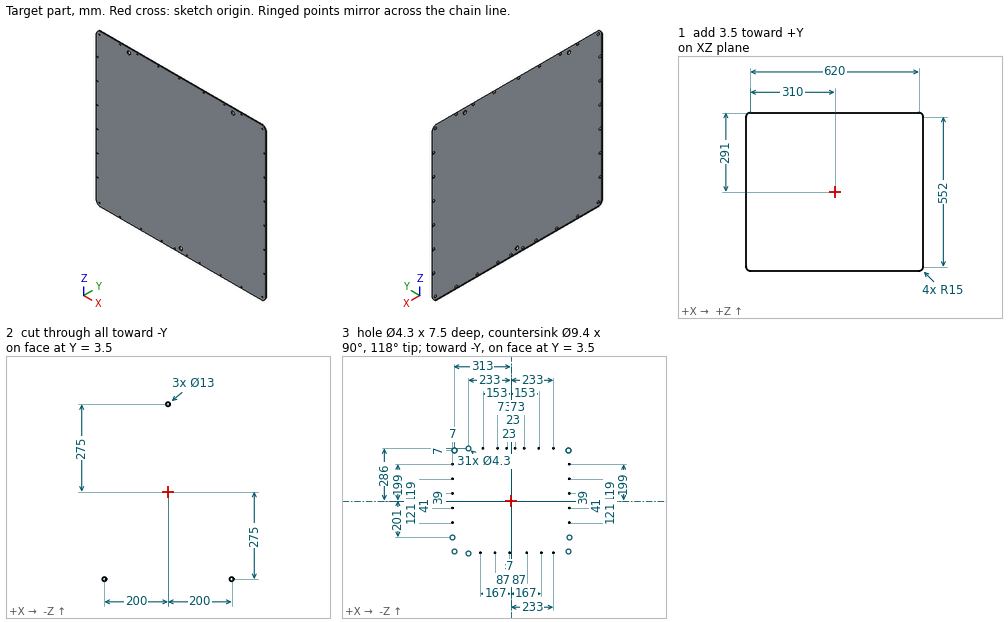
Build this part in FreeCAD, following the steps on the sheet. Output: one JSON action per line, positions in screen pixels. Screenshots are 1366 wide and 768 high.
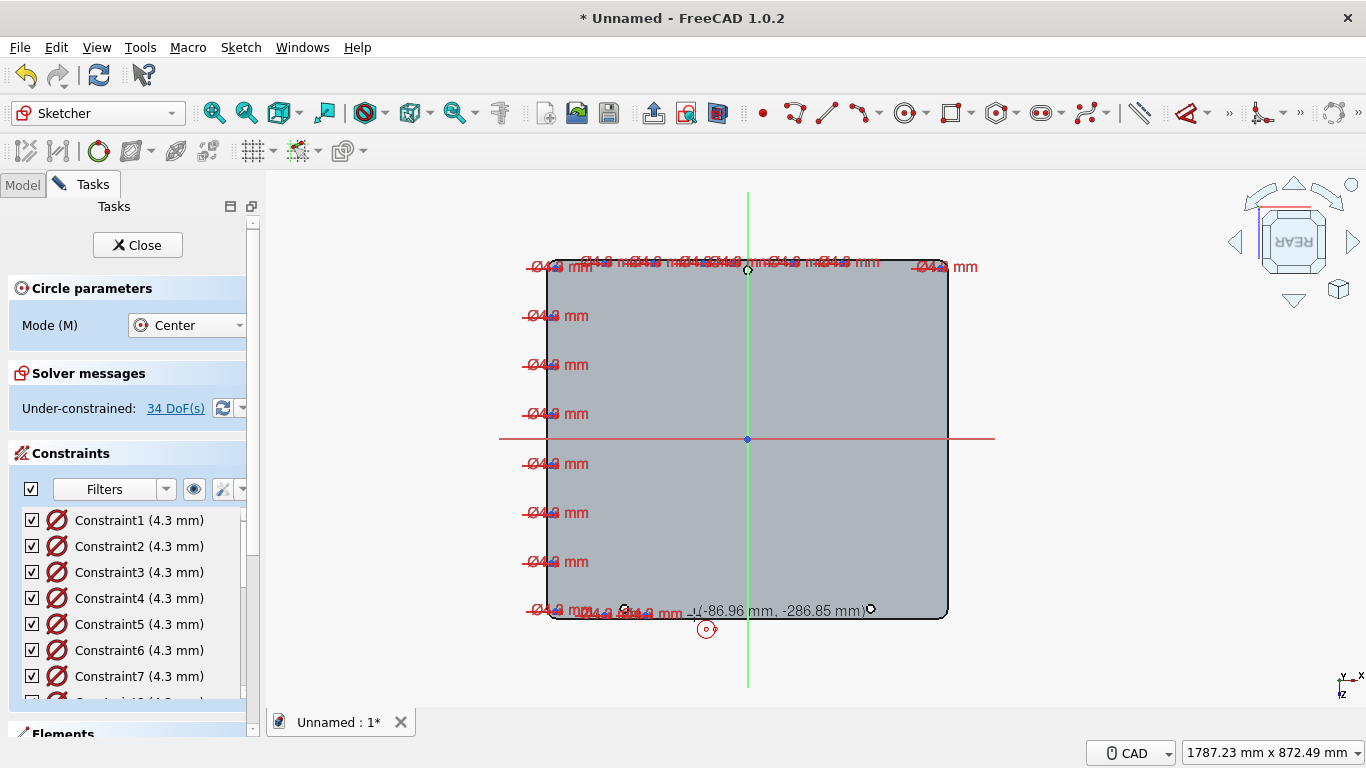
{"action": "left_click", "coordinate": [694, 615]}
{"action": "mouse_move", "coordinate": [695, 615]}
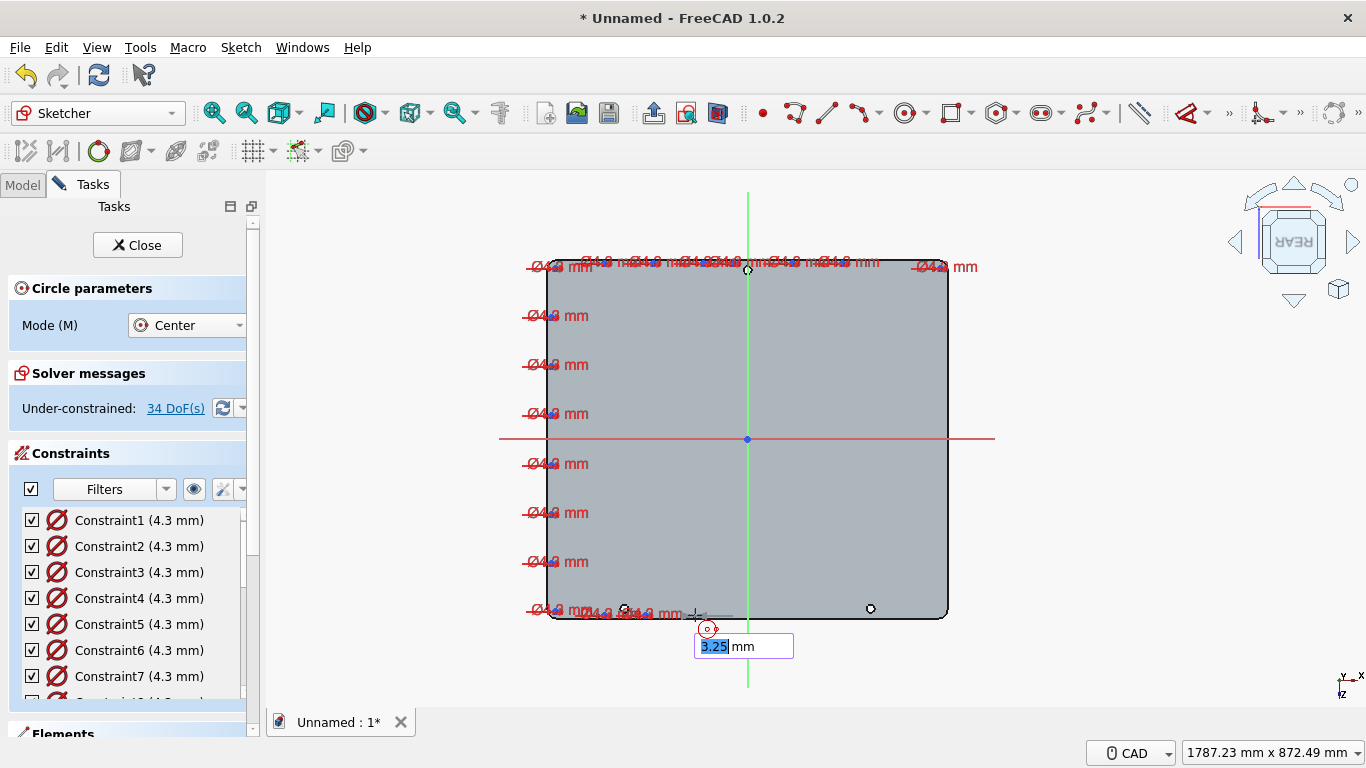
{"action": "type", "text": "4.3"}
{"action": "key", "text": "Return"}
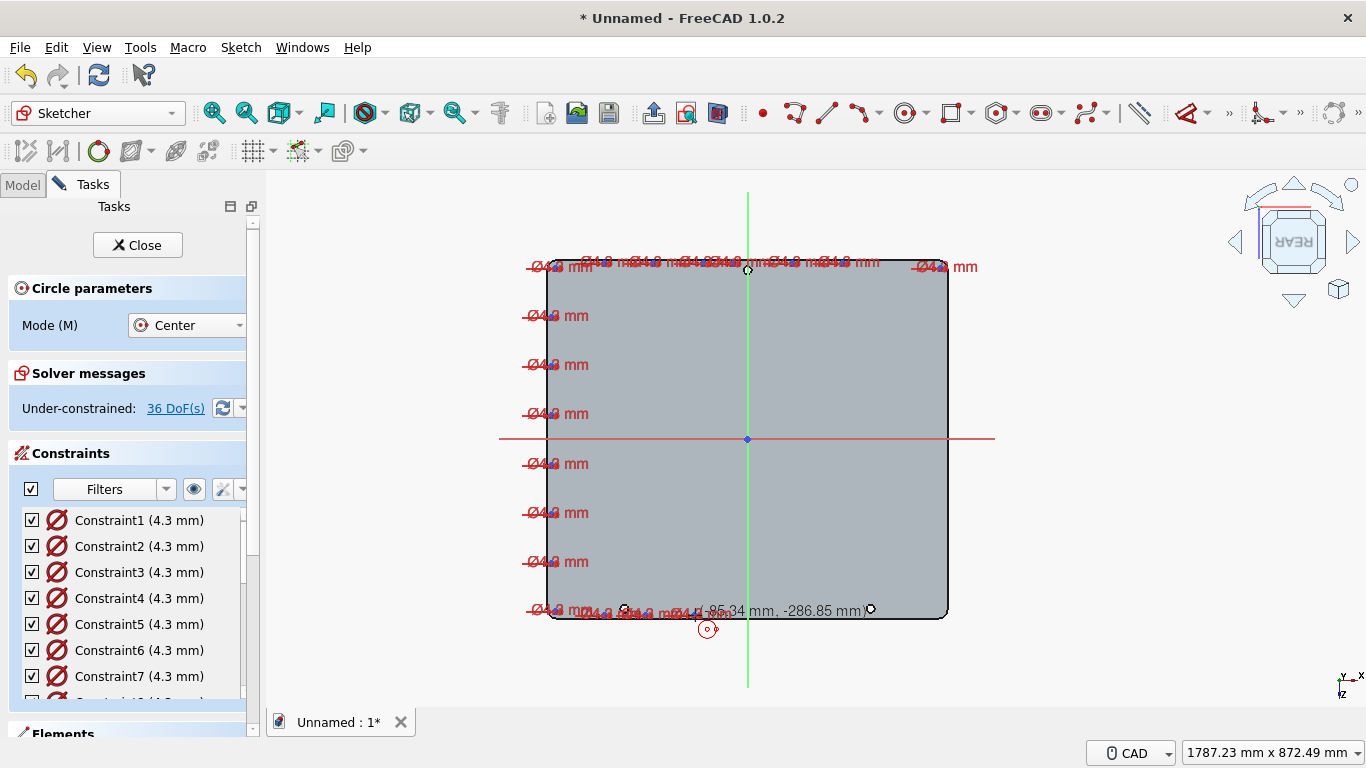
{"action": "scroll", "coordinate": [743, 615], "scroll_direction": "up", "scroll_amount": 15}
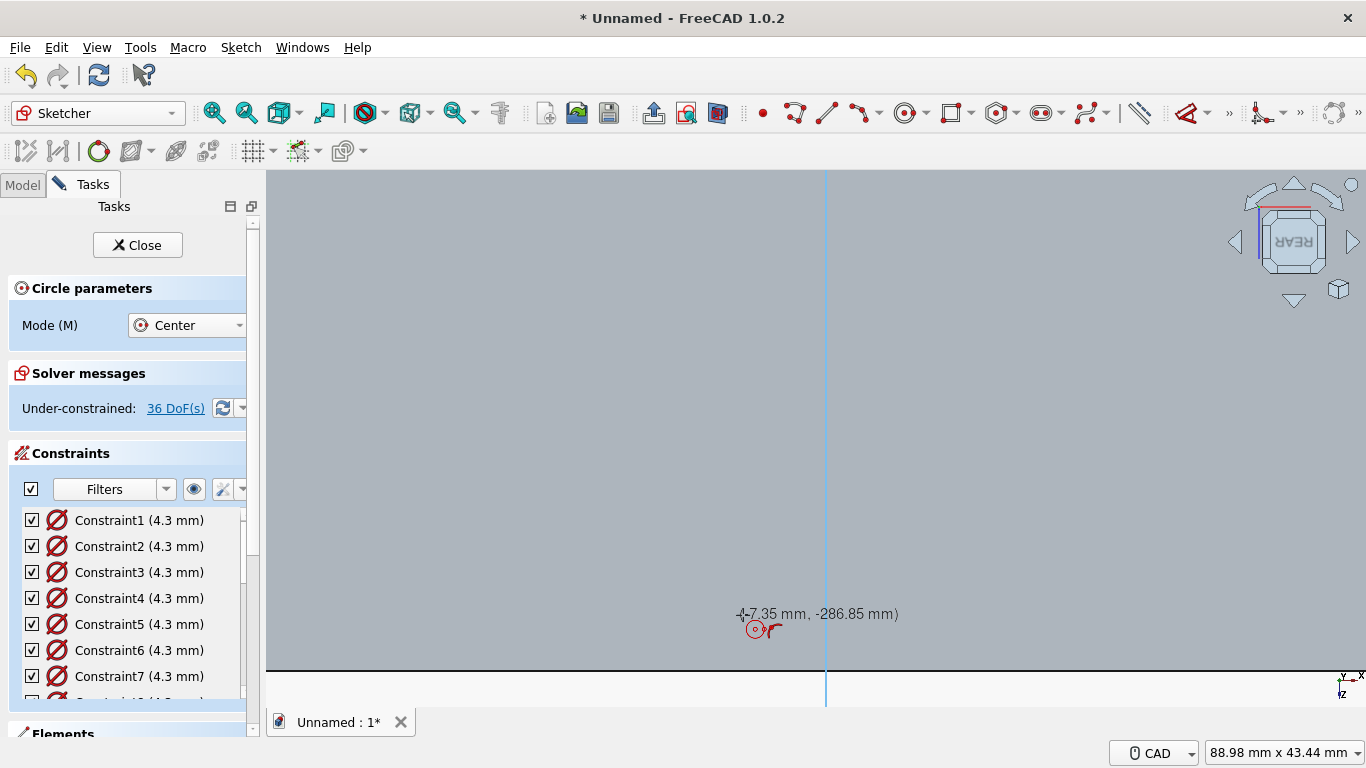
{"action": "scroll", "coordinate": [743, 615], "scroll_direction": "down", "scroll_amount": 15}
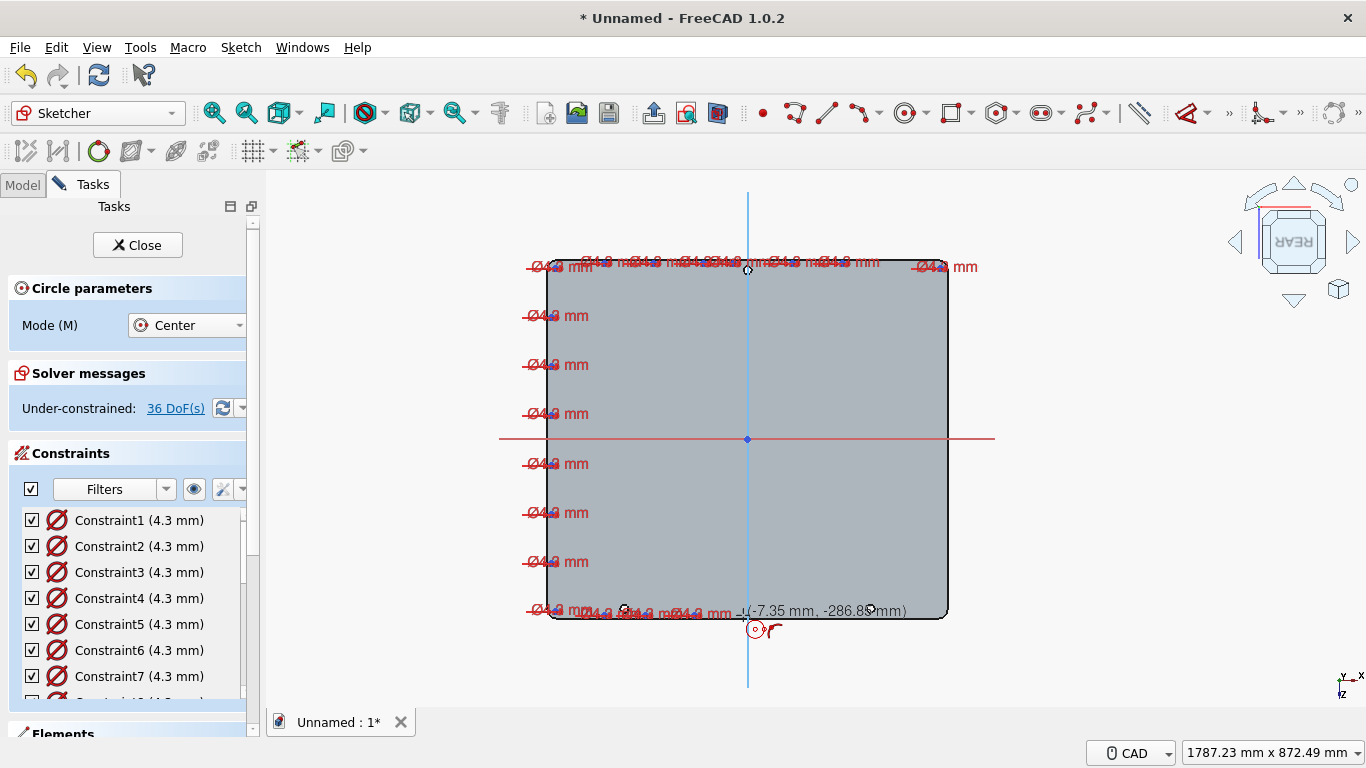
{"action": "scroll", "coordinate": [743, 615], "scroll_direction": "up", "scroll_amount": 7}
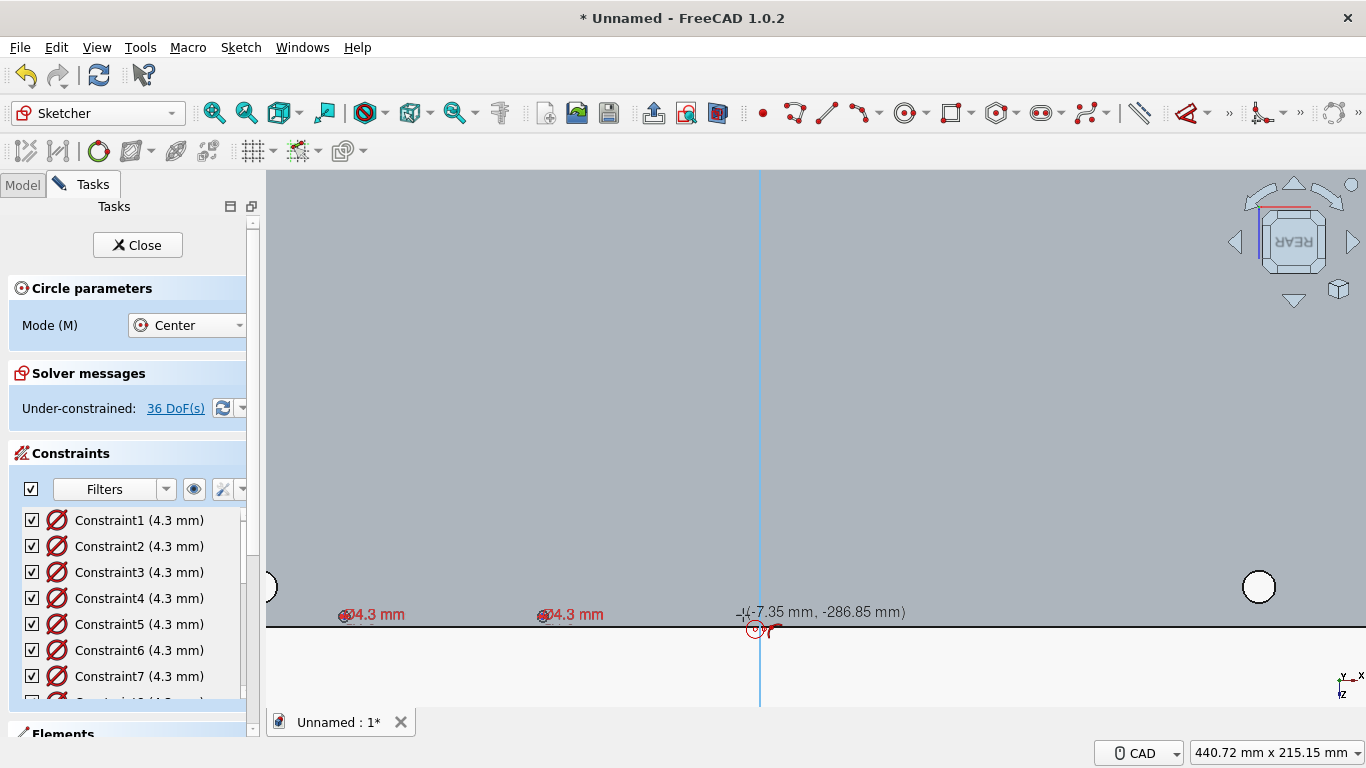
{"action": "left_click", "coordinate": [743, 614]}
{"action": "mouse_move", "coordinate": [739, 611]}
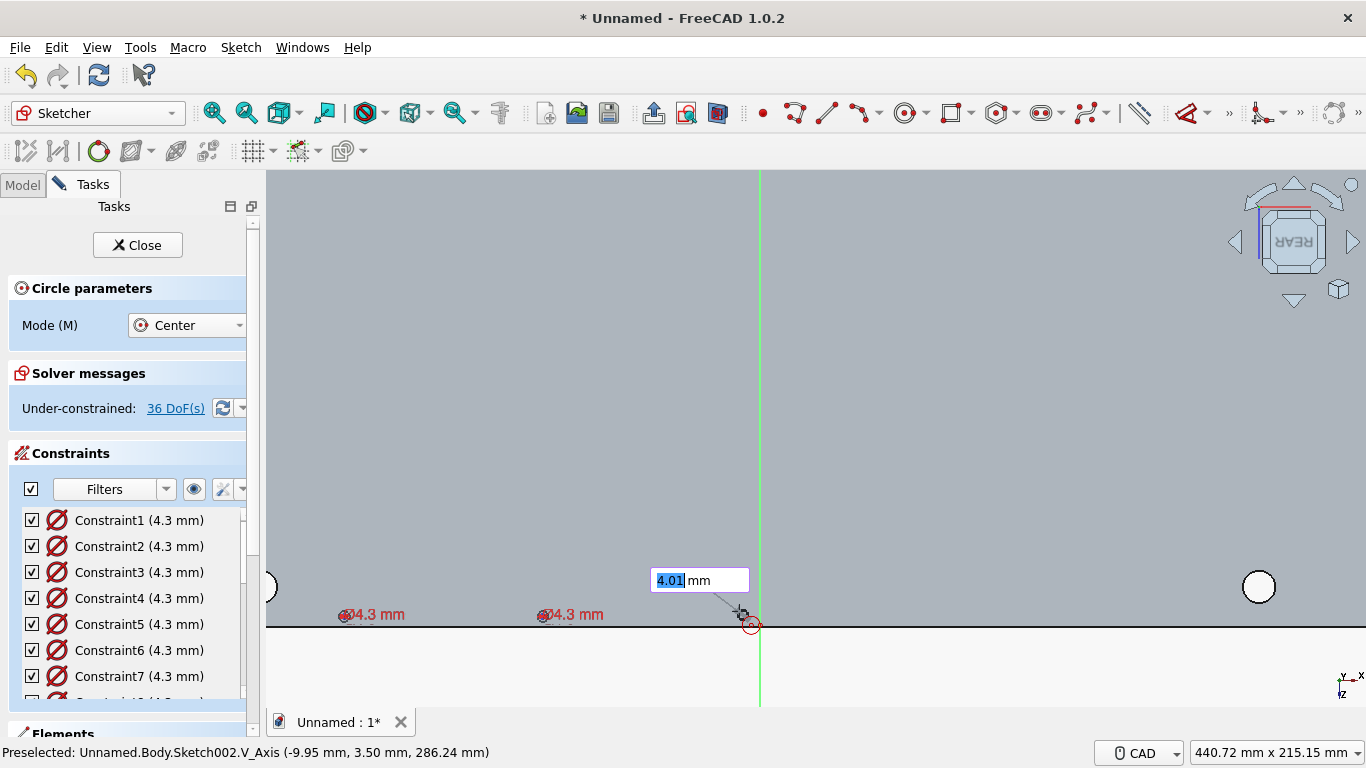
{"action": "type", "text": "4.3"}
{"action": "key", "text": "Return"}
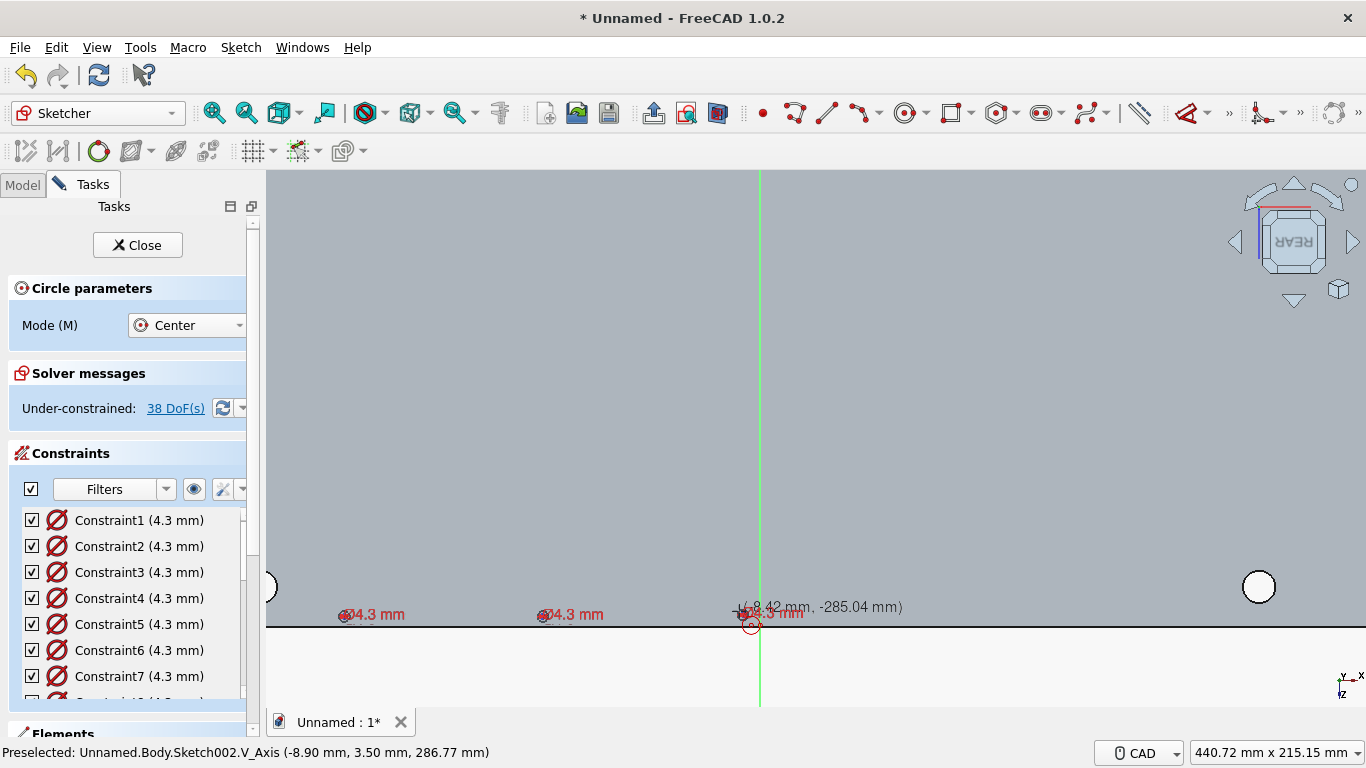
{"action": "scroll", "coordinate": [977, 614], "scroll_direction": "up", "scroll_amount": 8}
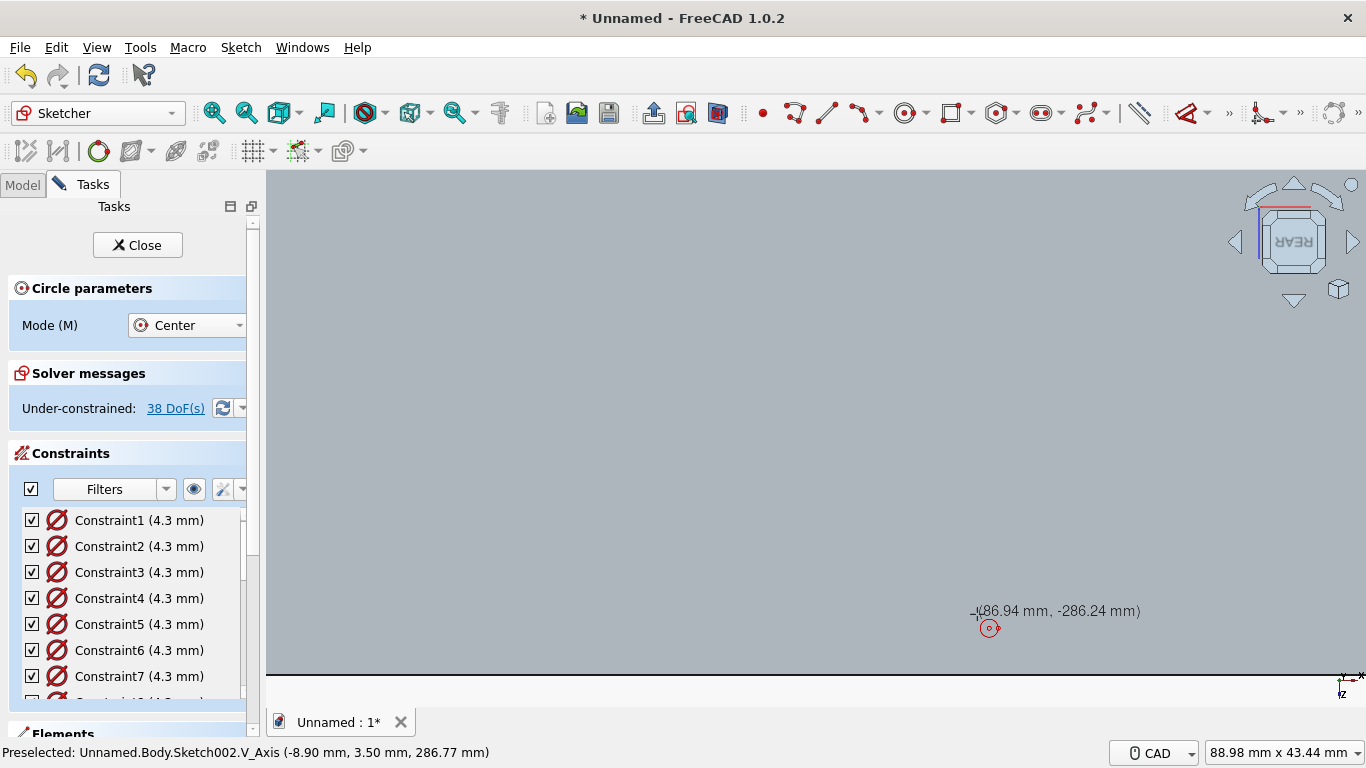
{"action": "scroll", "coordinate": [792, 615], "scroll_direction": "down", "scroll_amount": 15}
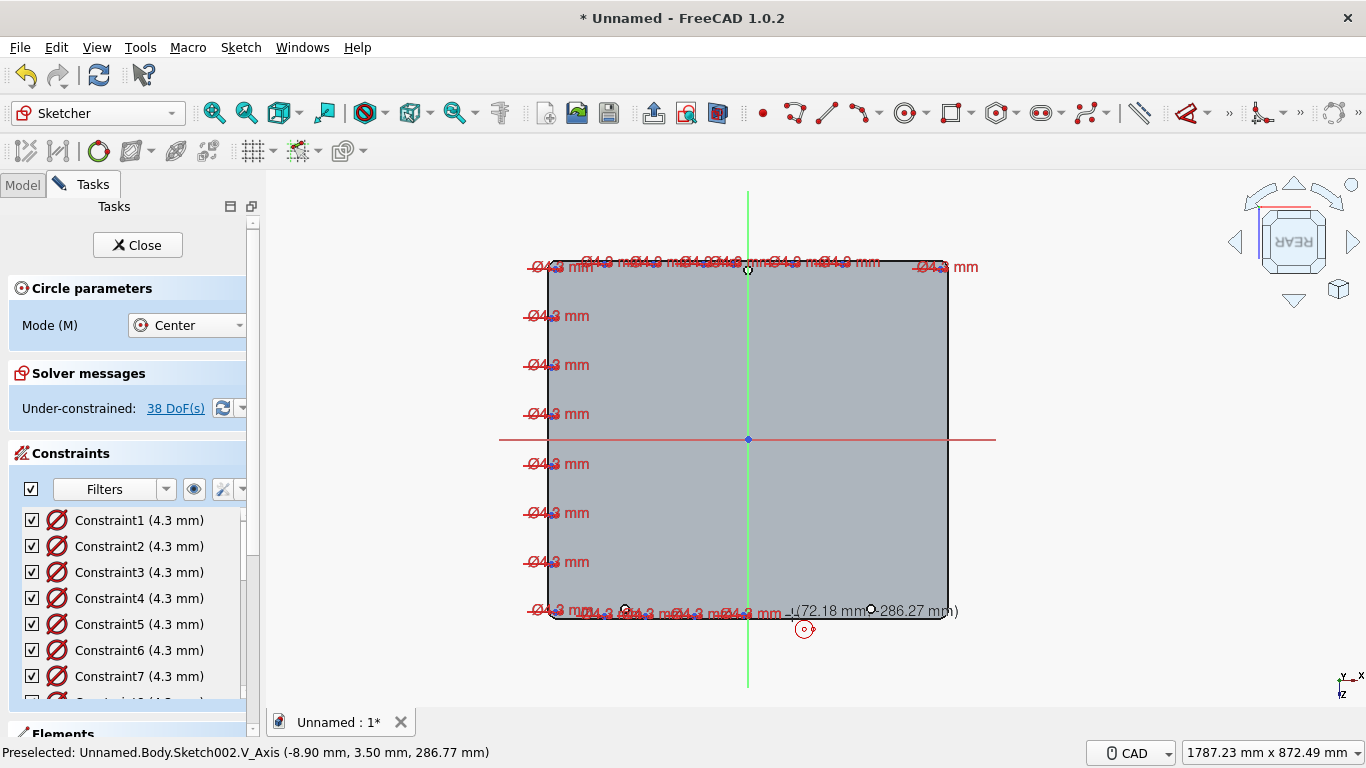
{"action": "left_click", "coordinate": [802, 616]}
{"action": "mouse_move", "coordinate": [803, 615]}